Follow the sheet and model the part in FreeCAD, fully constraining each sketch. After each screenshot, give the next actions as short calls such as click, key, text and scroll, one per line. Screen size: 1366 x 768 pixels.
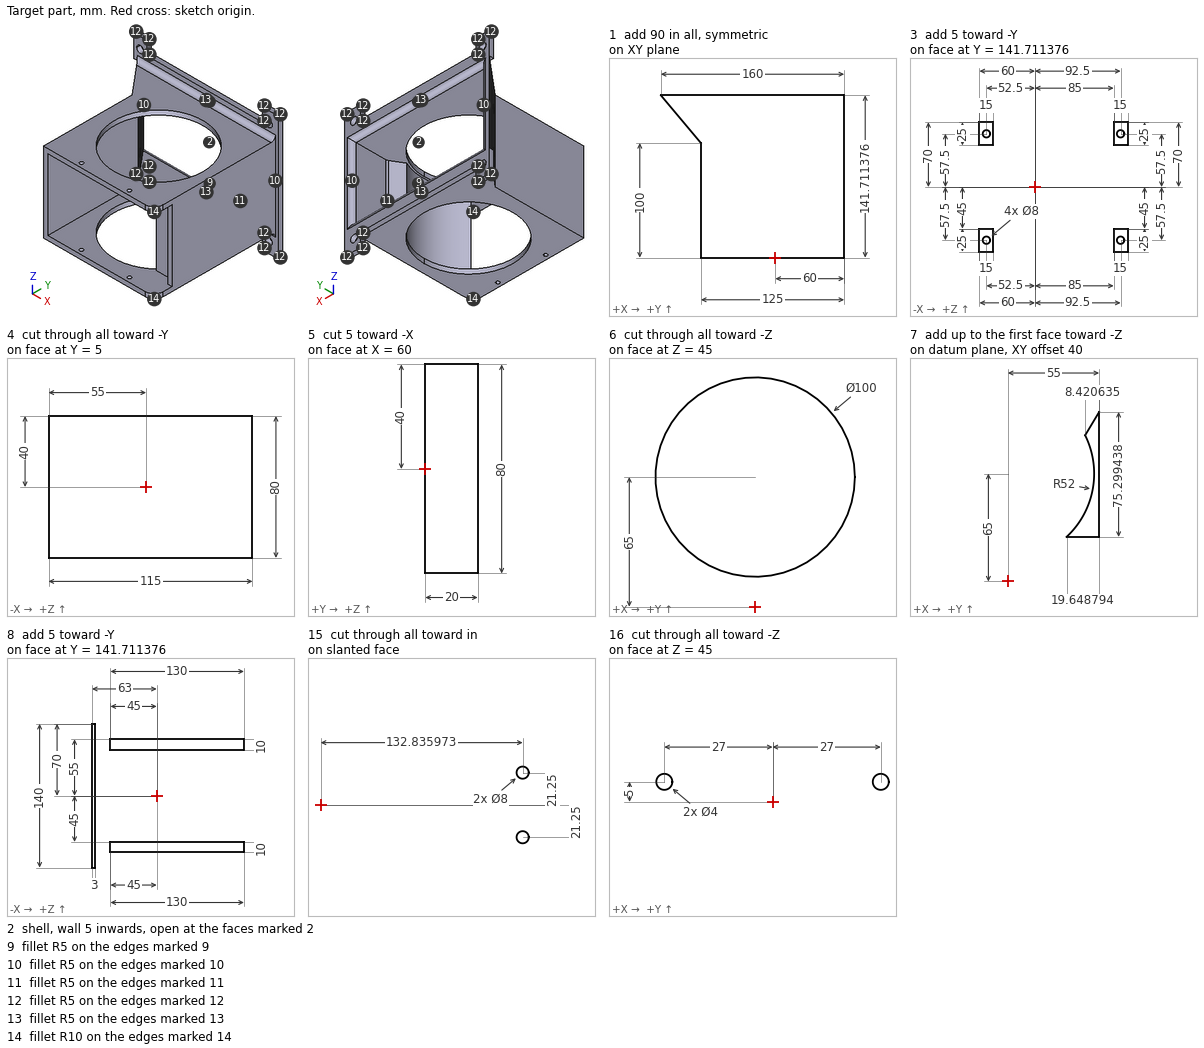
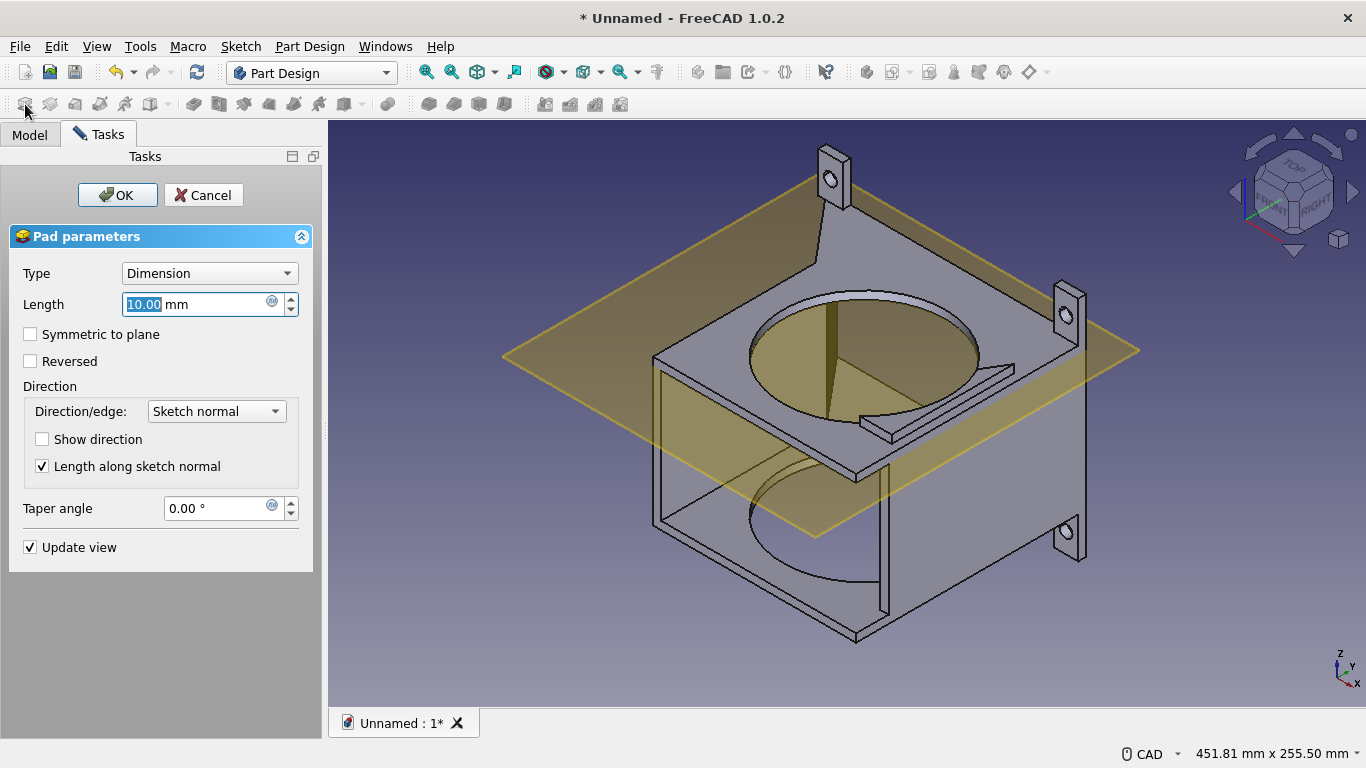
click(210, 274)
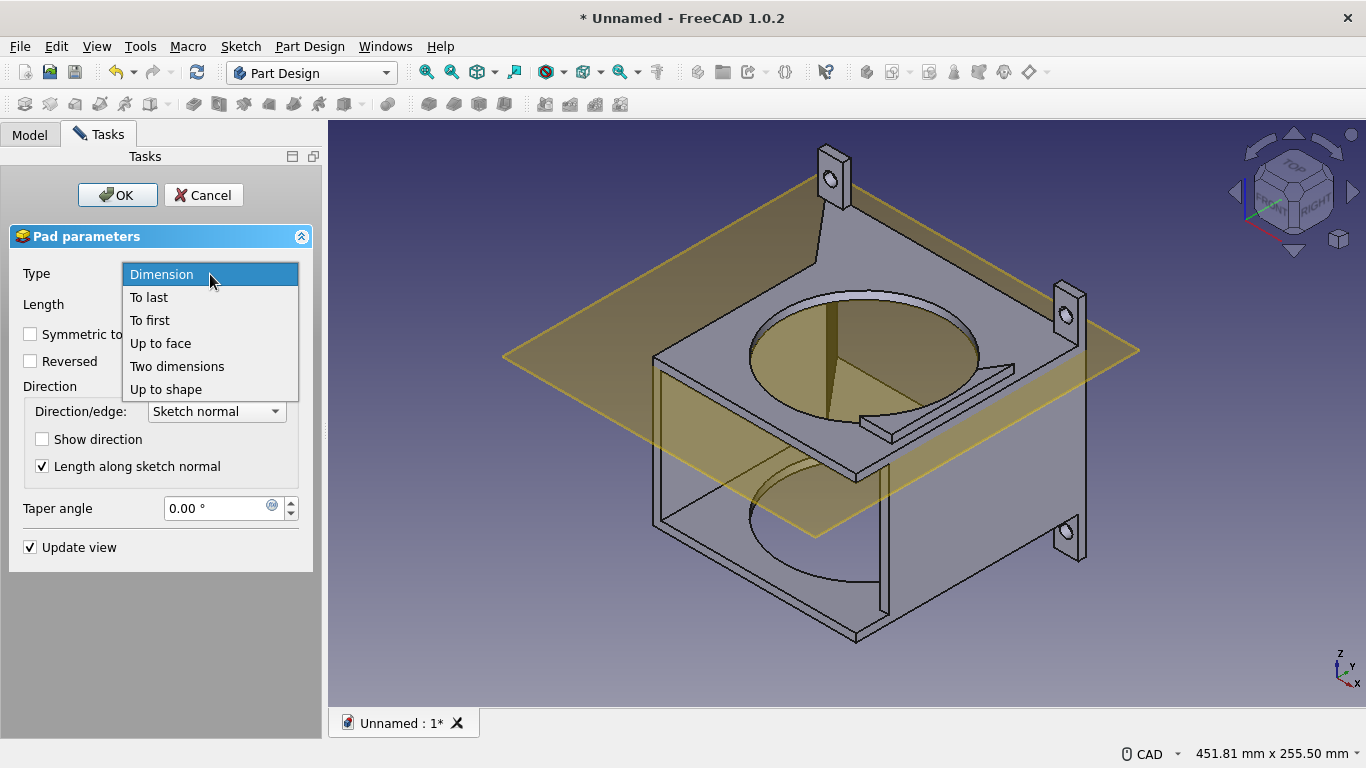
click(208, 320)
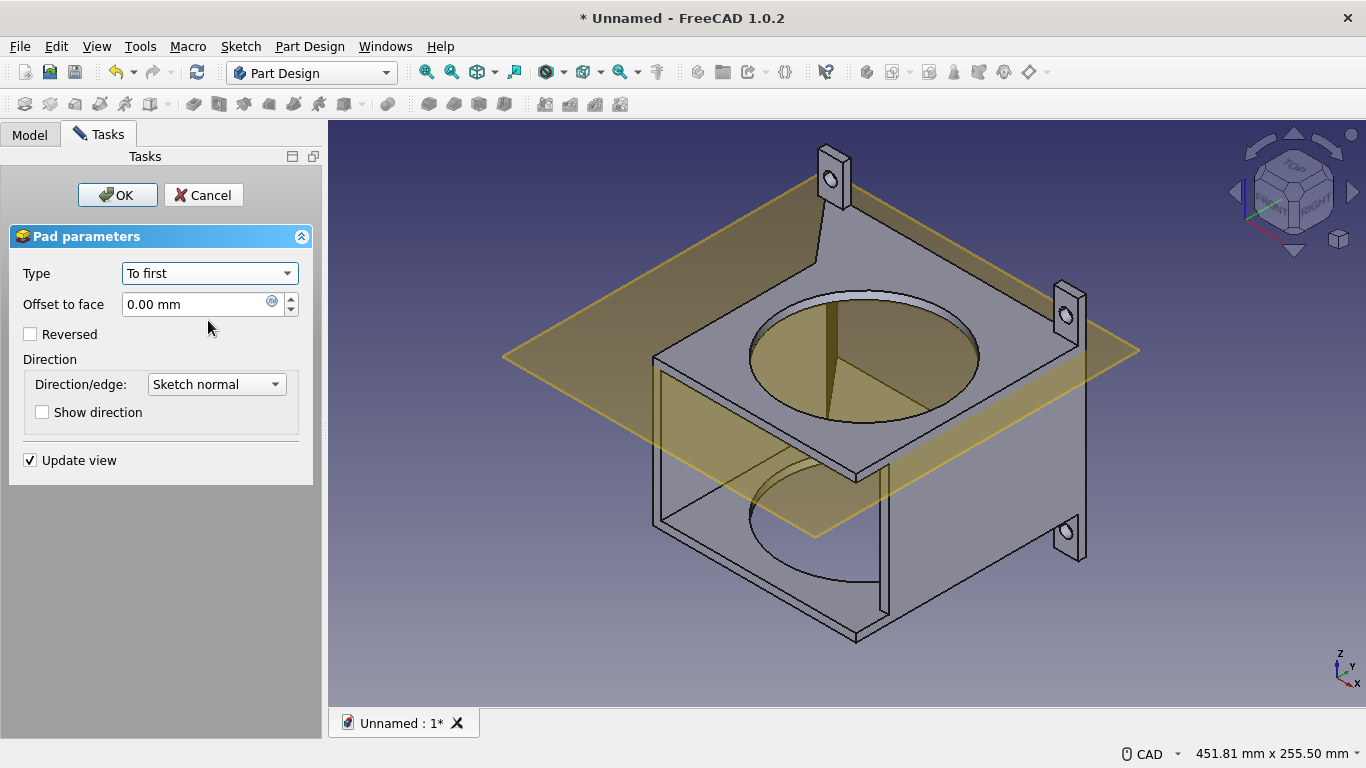
click(31, 334)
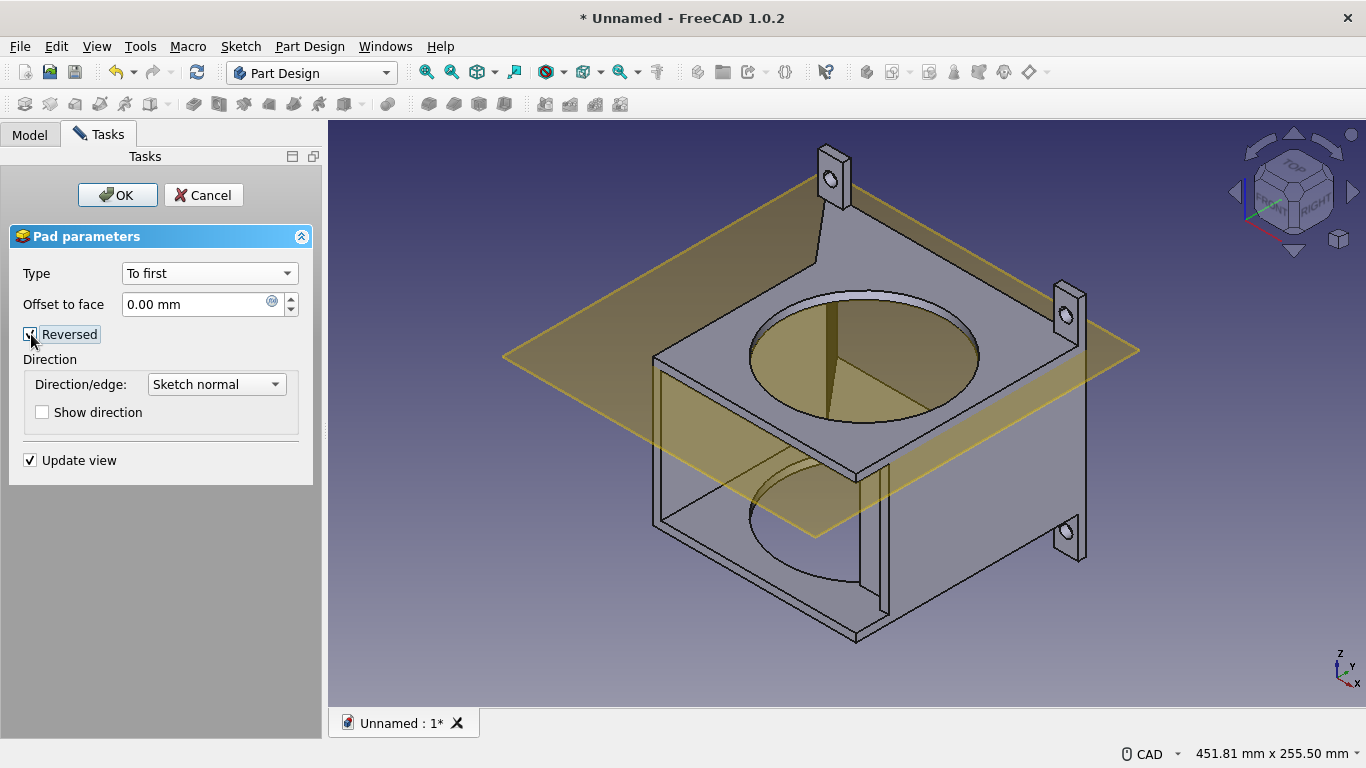
click(118, 195)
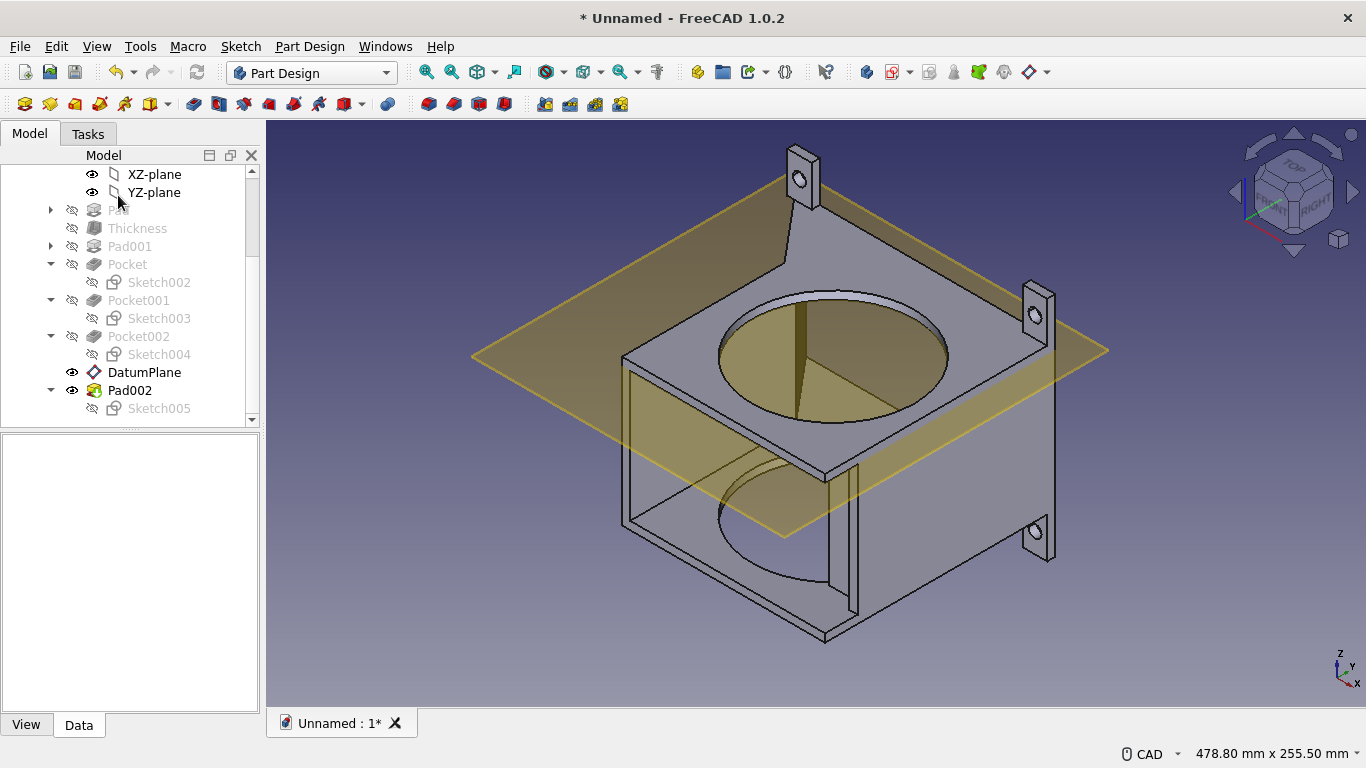
click(117, 372)
key(space)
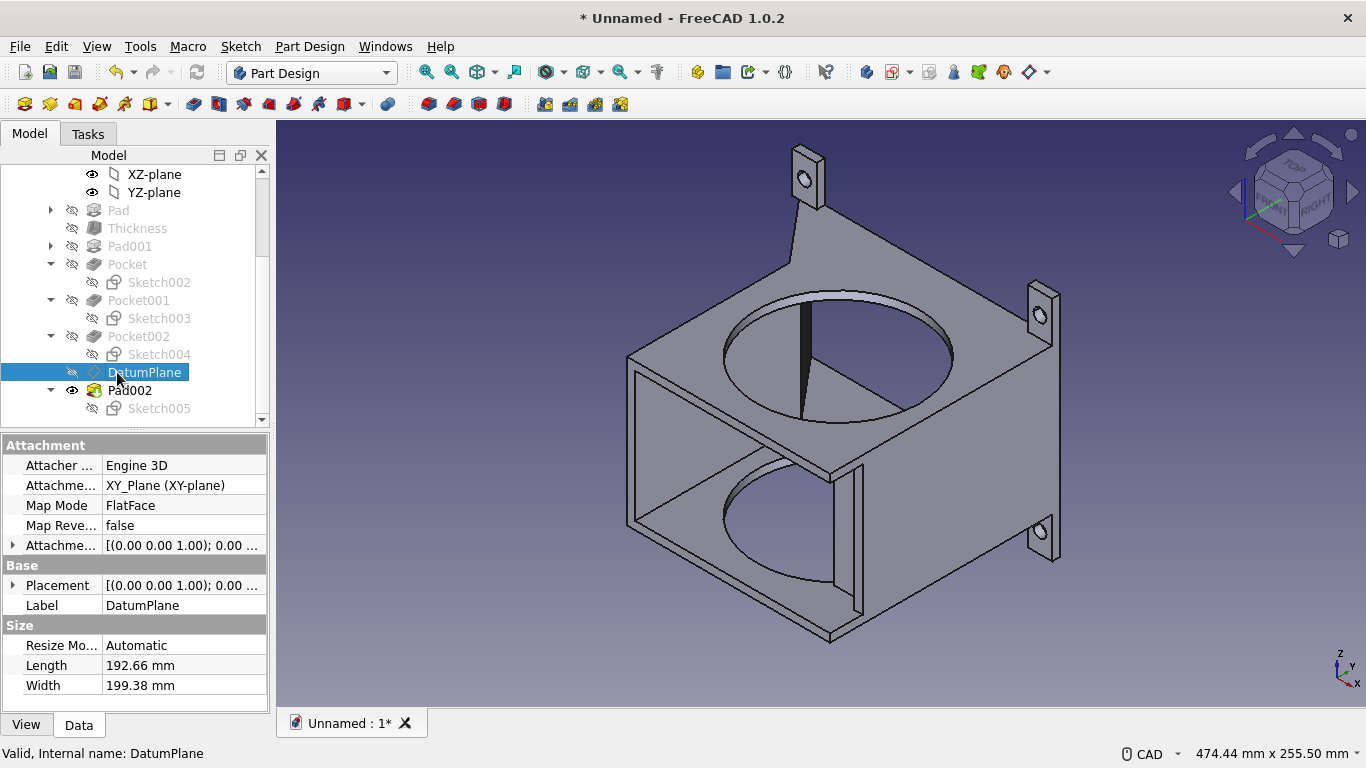
key(4)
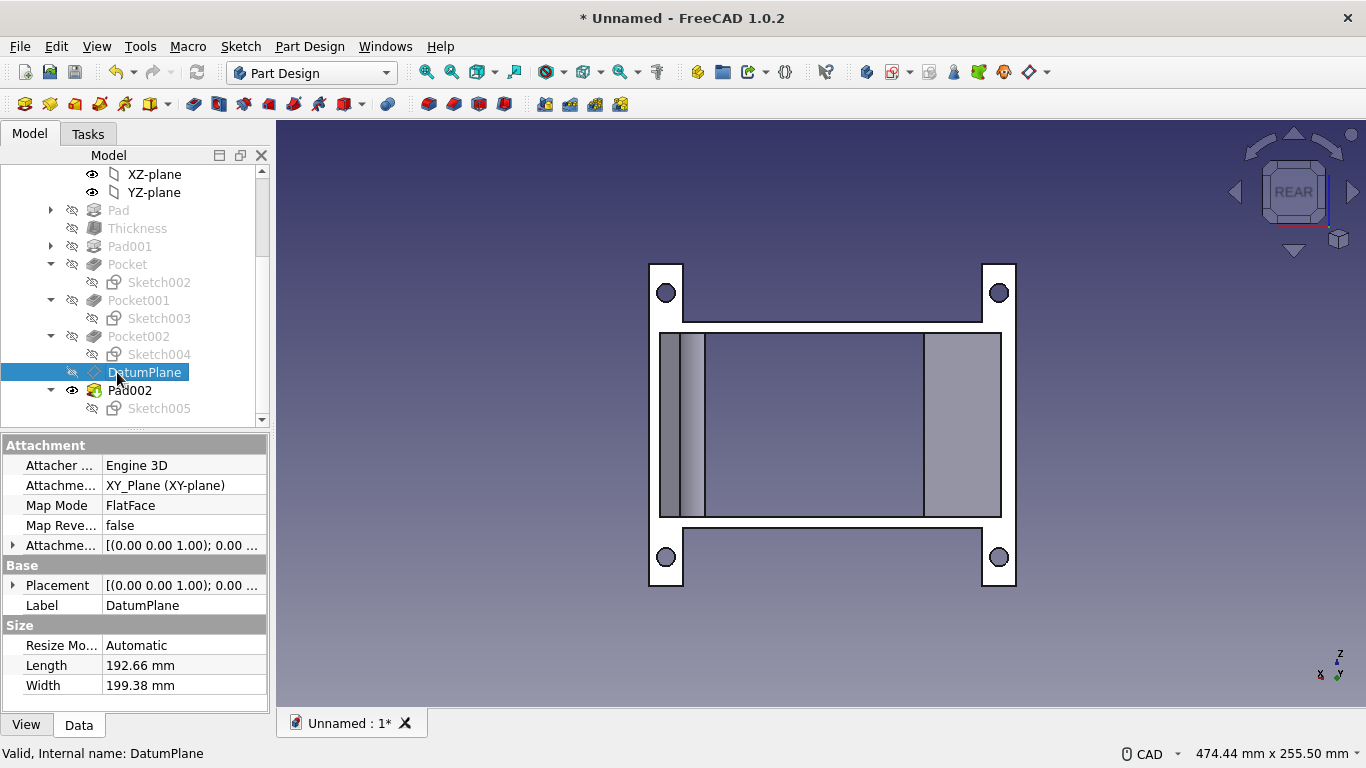
scroll(990, 286, up, 11)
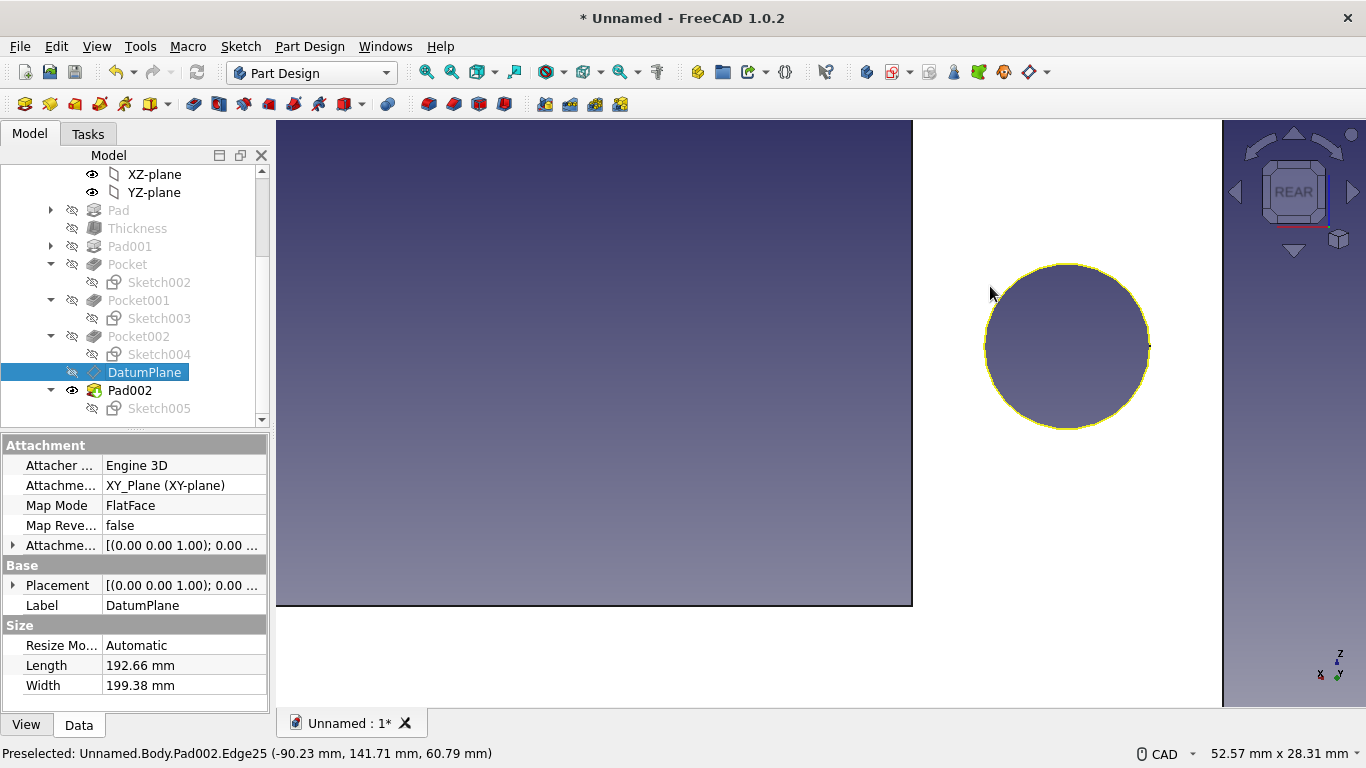
click(986, 294)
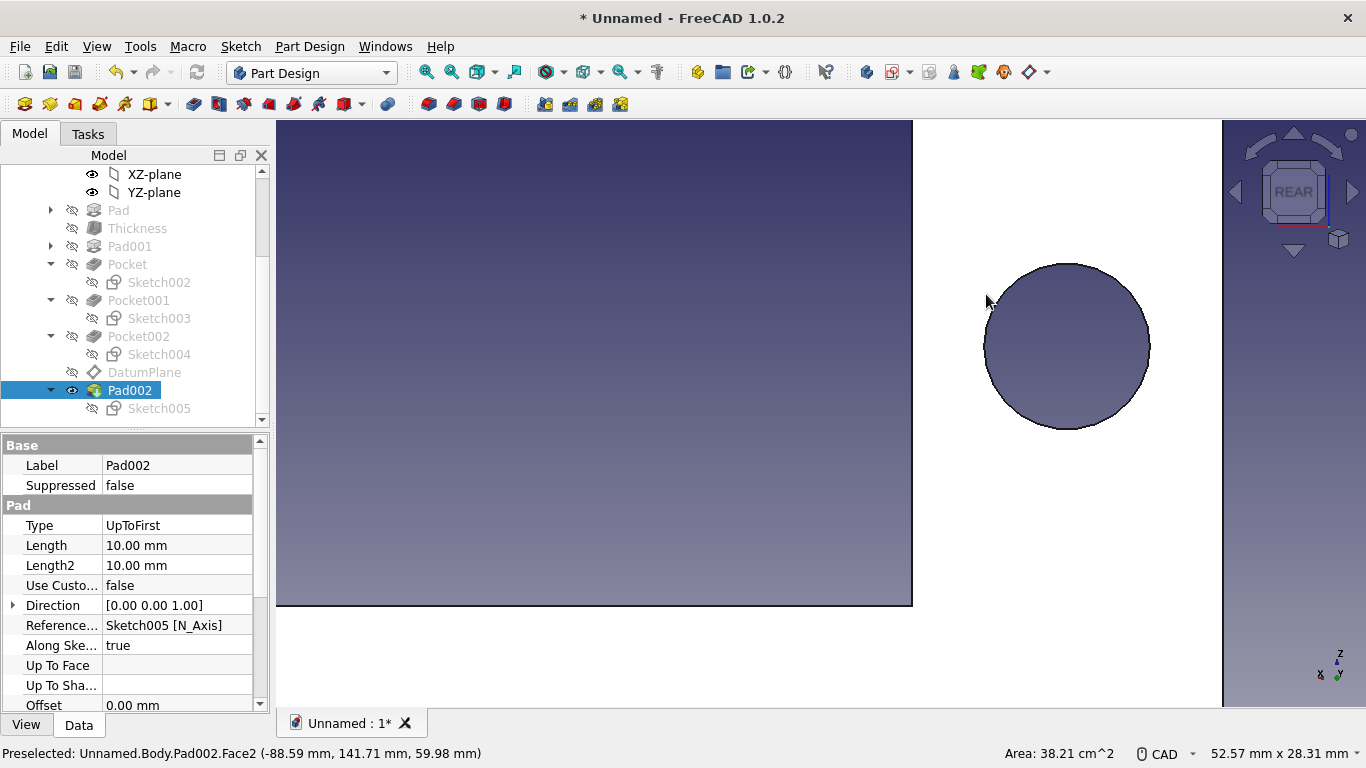
click(892, 72)